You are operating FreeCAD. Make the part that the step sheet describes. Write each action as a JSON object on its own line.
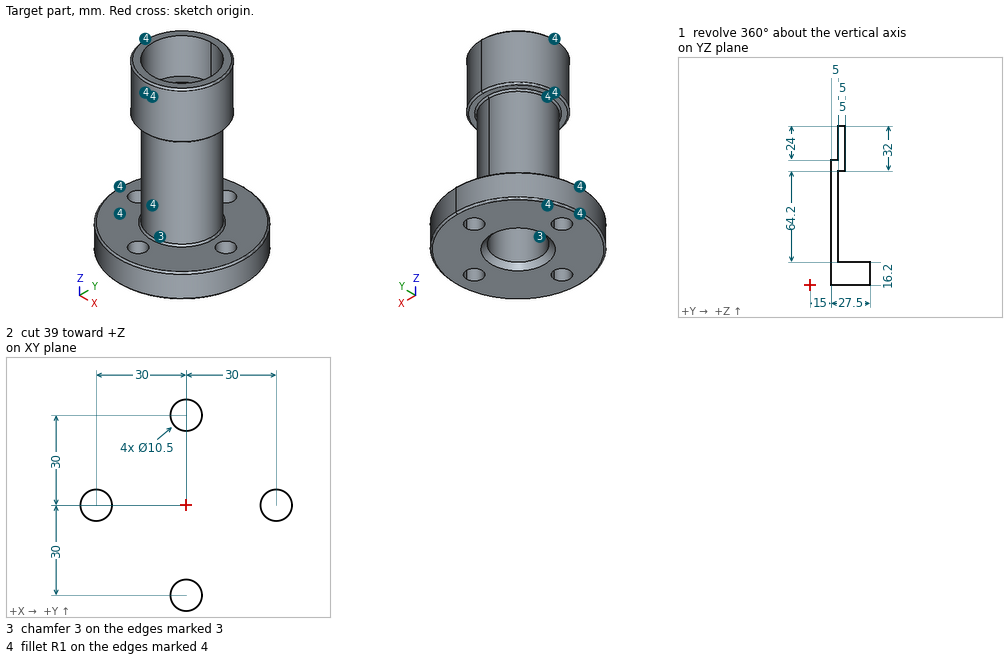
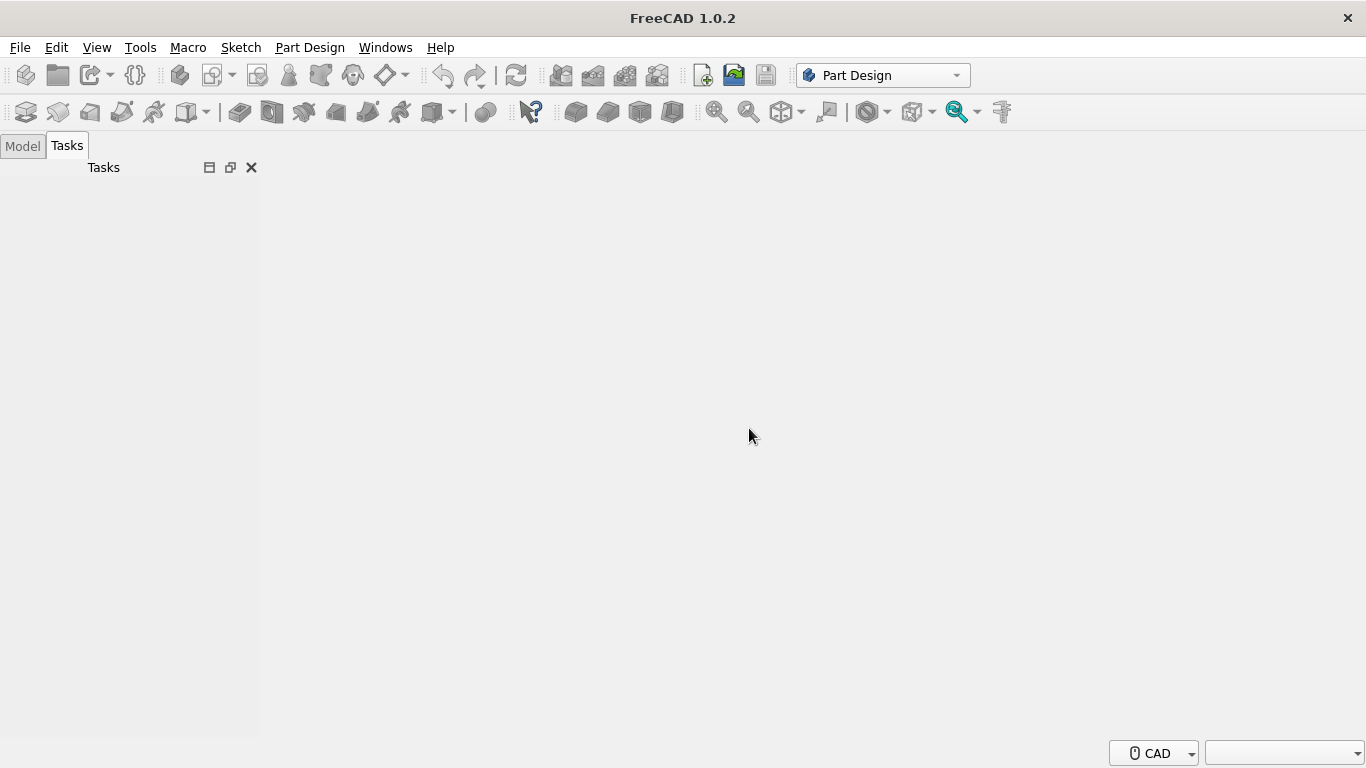
{"action": "left_click", "coordinate": [702, 76]}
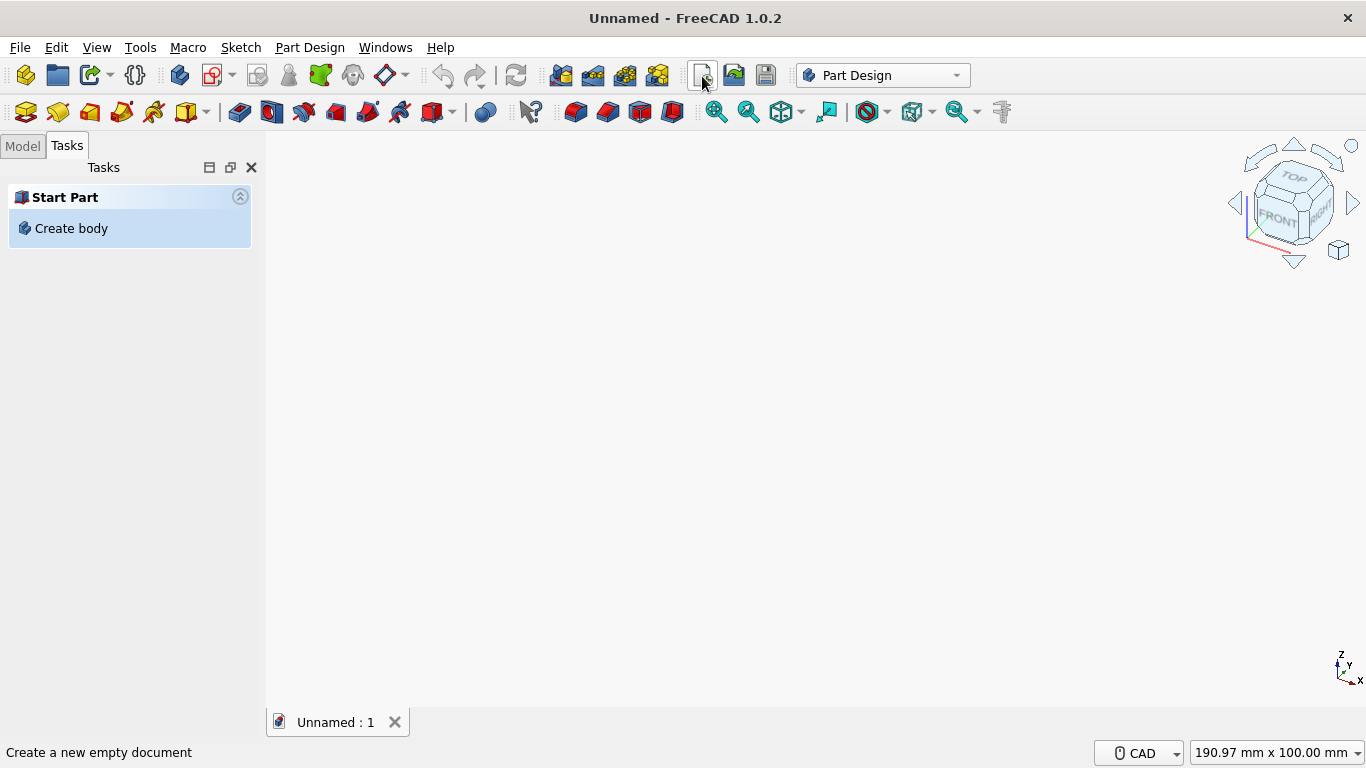
{"action": "left_click", "coordinate": [212, 76]}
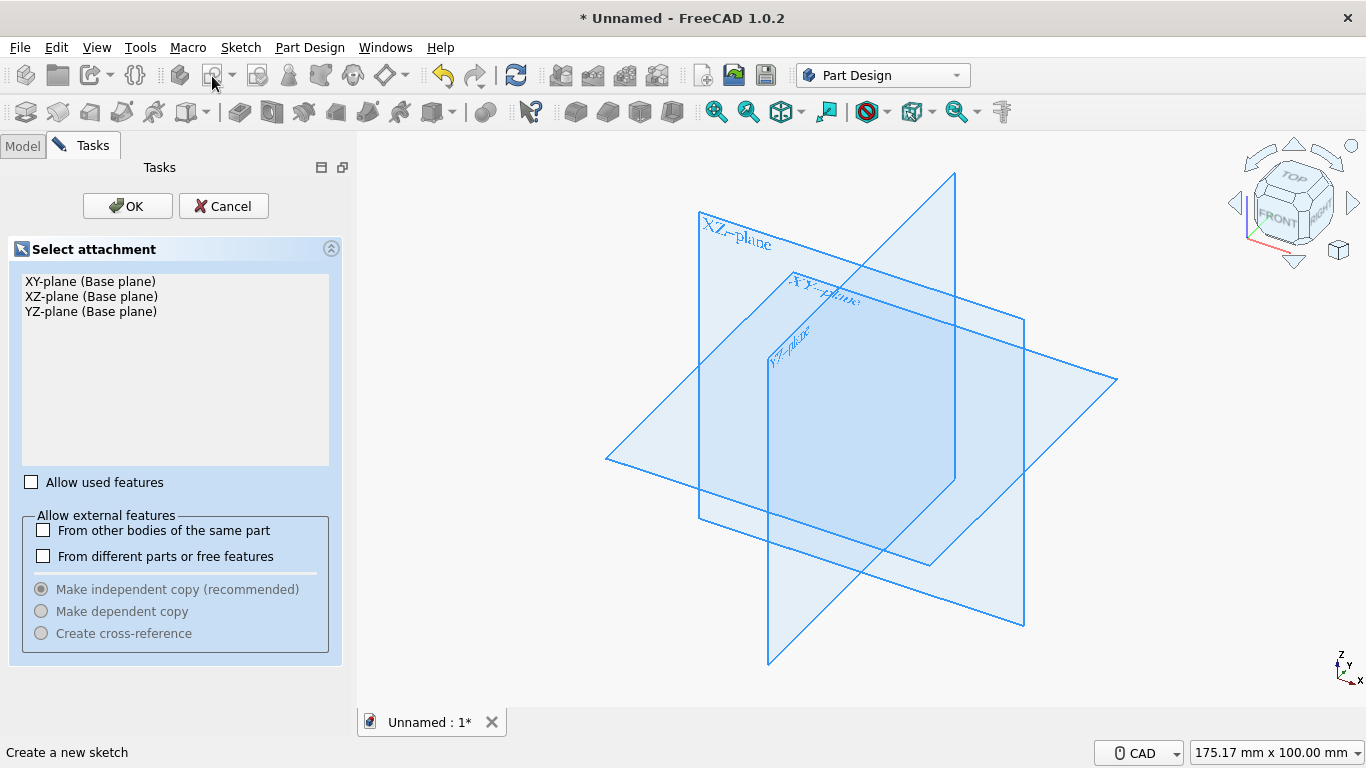
{"action": "left_click", "coordinate": [82, 312]}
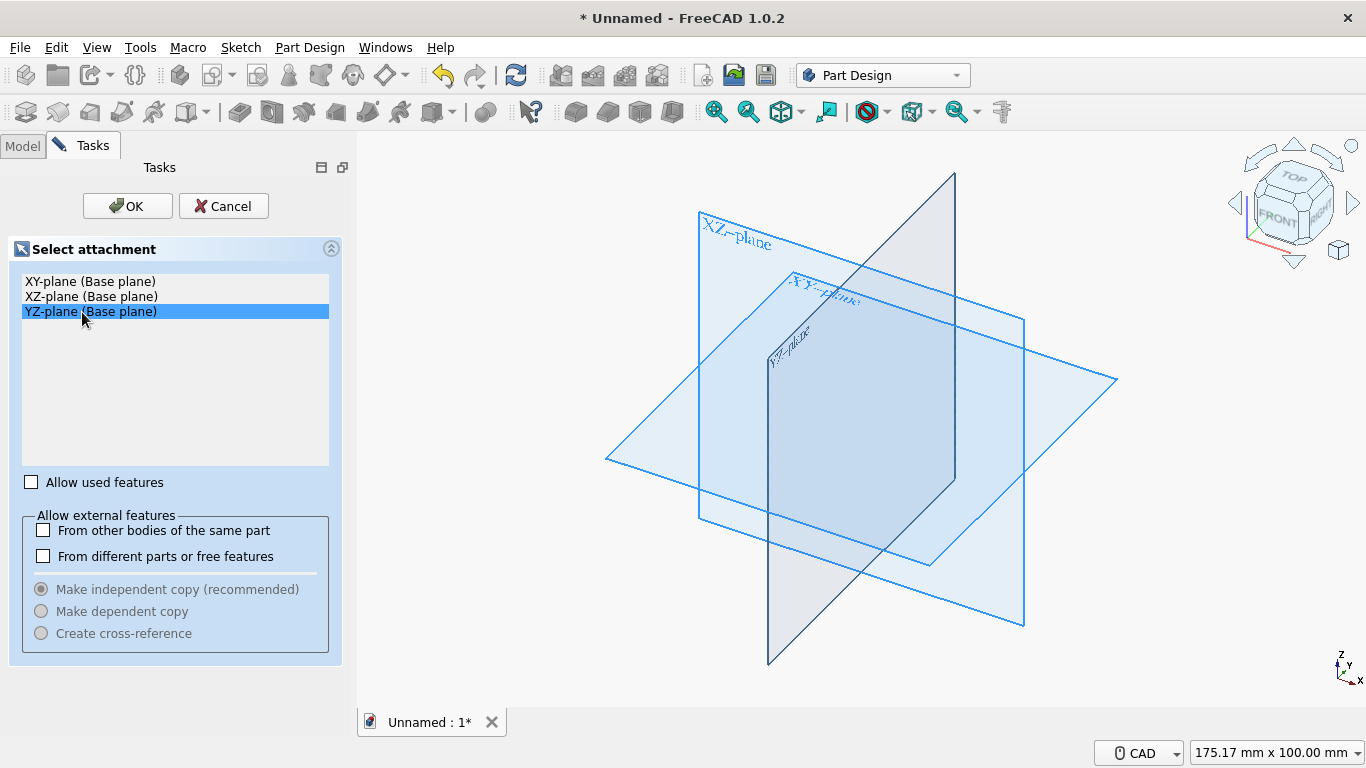
{"action": "left_click", "coordinate": [128, 206]}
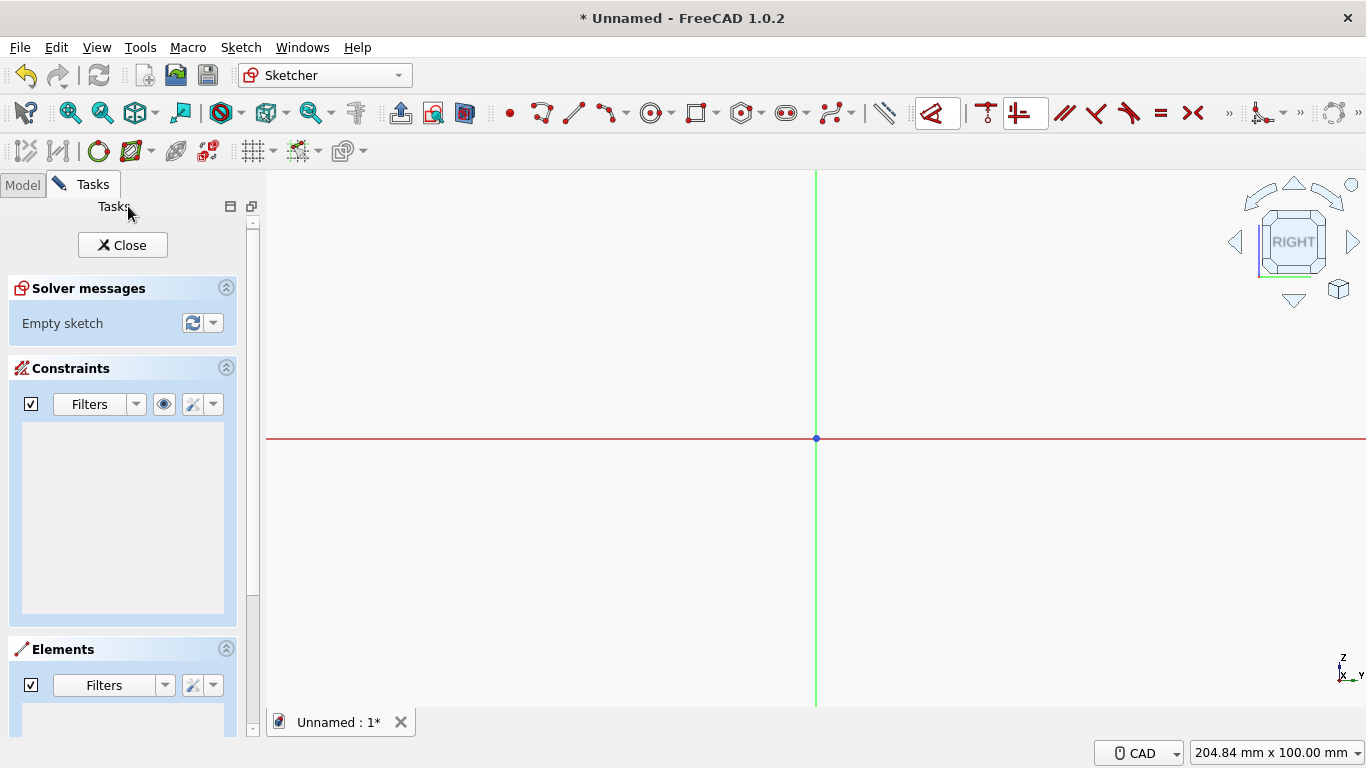
{"action": "scroll", "coordinate": [598, 679], "scroll_direction": "down", "scroll_amount": 4}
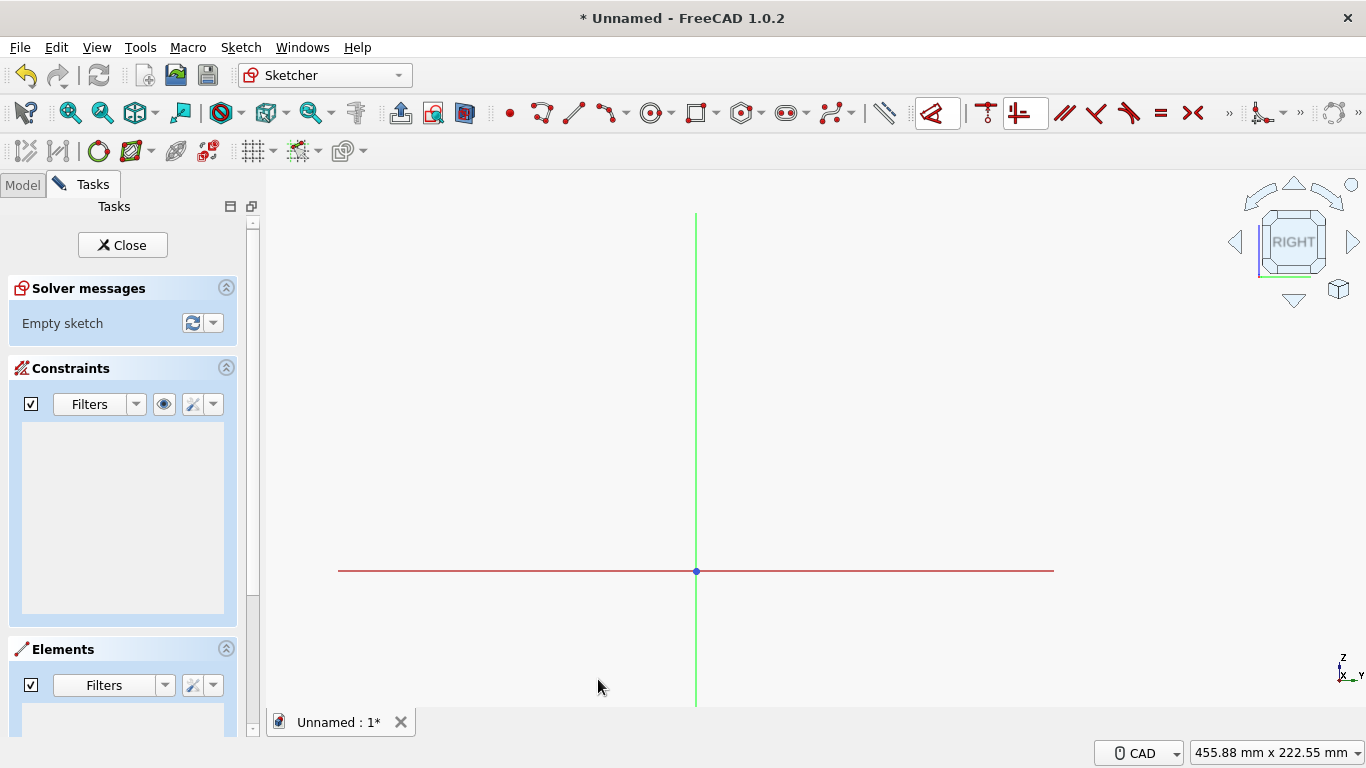
{"action": "left_click", "coordinate": [542, 114]}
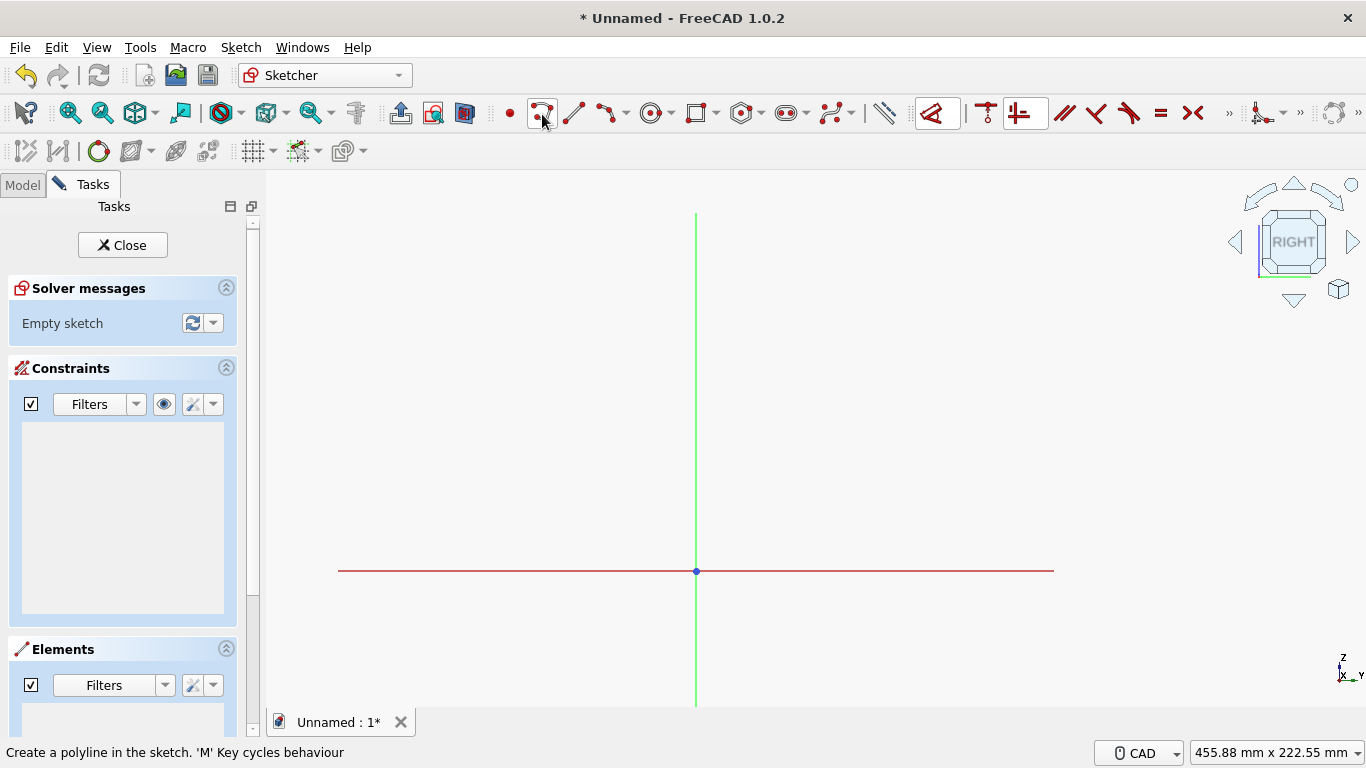
{"action": "left_click", "coordinate": [732, 571]}
{"action": "left_click", "coordinate": [799, 562]}
{"action": "left_click", "coordinate": [799, 532]}
{"action": "left_click", "coordinate": [744, 532]}
{"action": "left_click", "coordinate": [744, 377]}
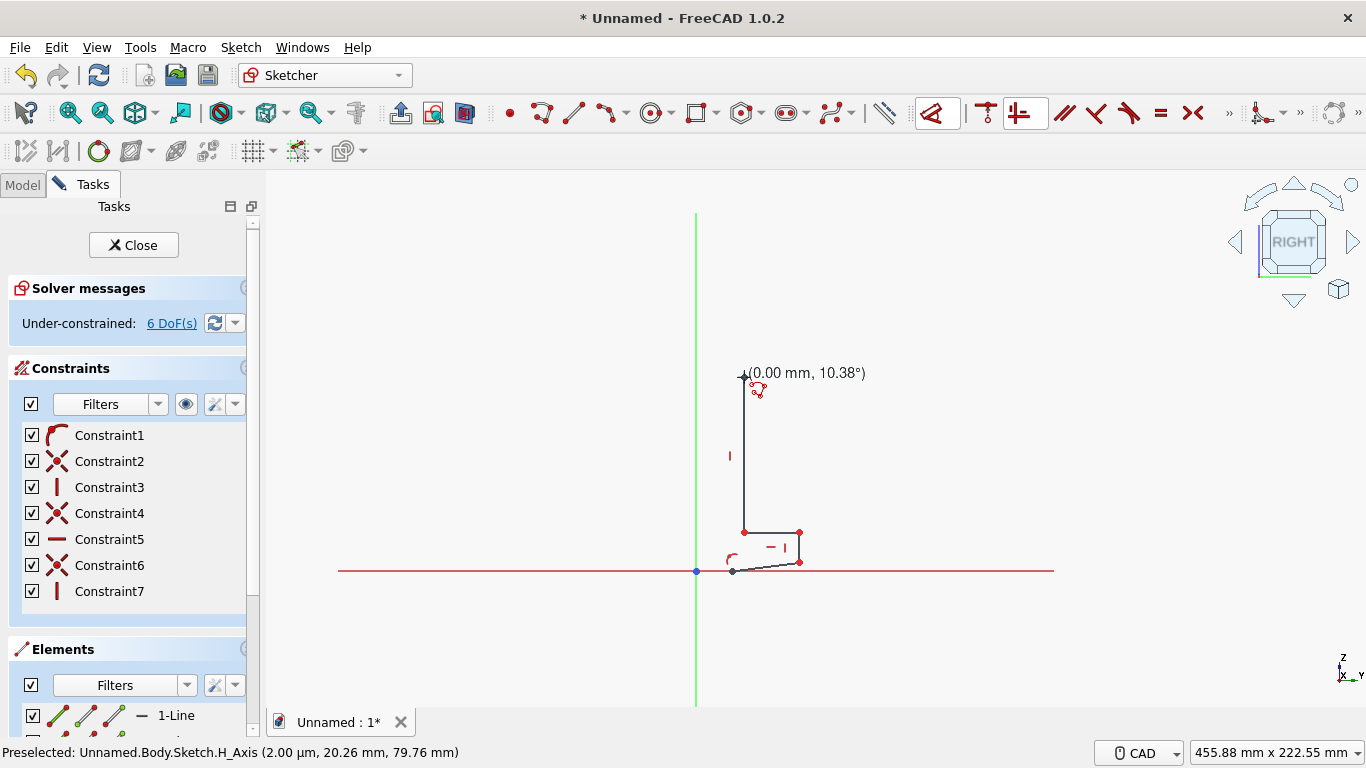
{"action": "scroll", "coordinate": [756, 377], "scroll_direction": "up", "scroll_amount": 2}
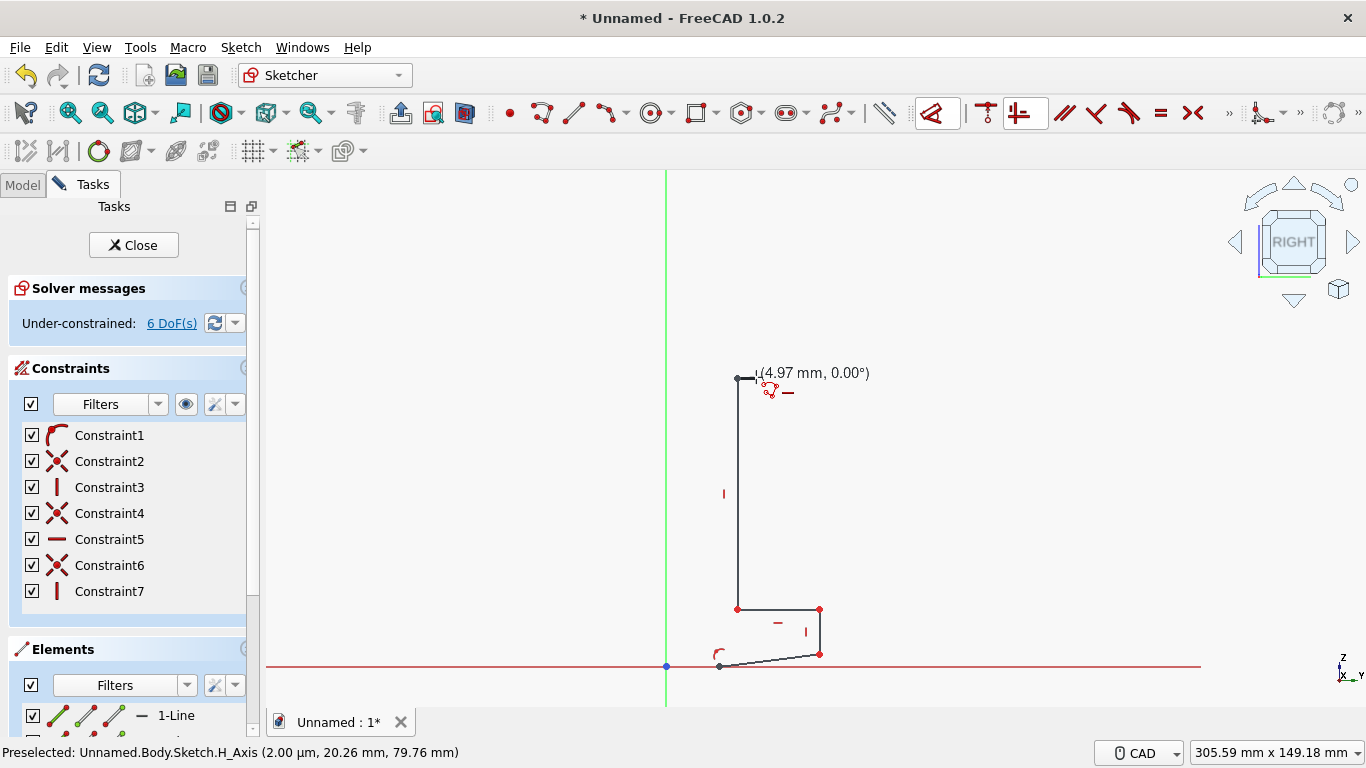
{"action": "left_click", "coordinate": [756, 377]}
{"action": "left_click", "coordinate": [756, 262]}
{"action": "left_click", "coordinate": [738, 262]}
{"action": "left_click", "coordinate": [738, 349]}
{"action": "left_click", "coordinate": [720, 349]}
{"action": "left_click", "coordinate": [720, 667]}
{"action": "key", "text": "Escape"}
{"action": "key", "text": "Escape"}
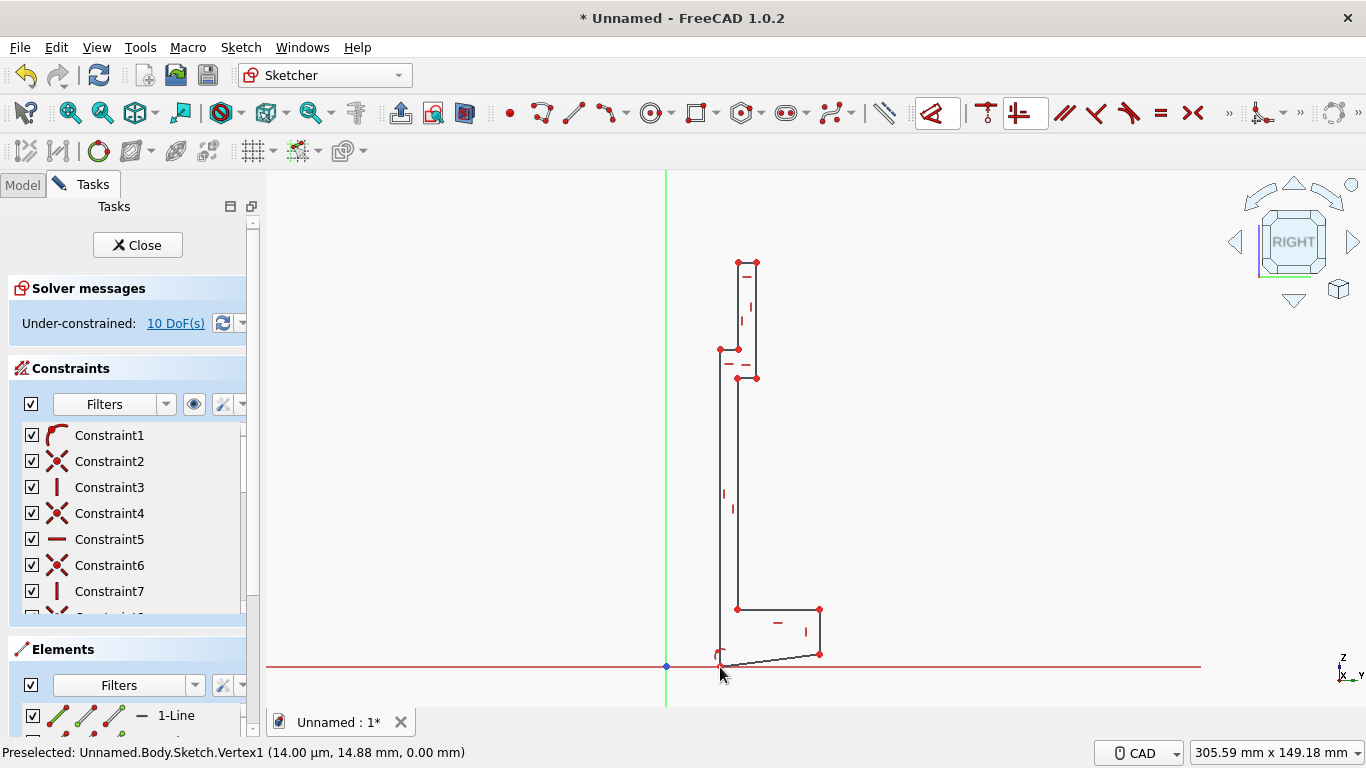
{"action": "left_click", "coordinate": [750, 663]}